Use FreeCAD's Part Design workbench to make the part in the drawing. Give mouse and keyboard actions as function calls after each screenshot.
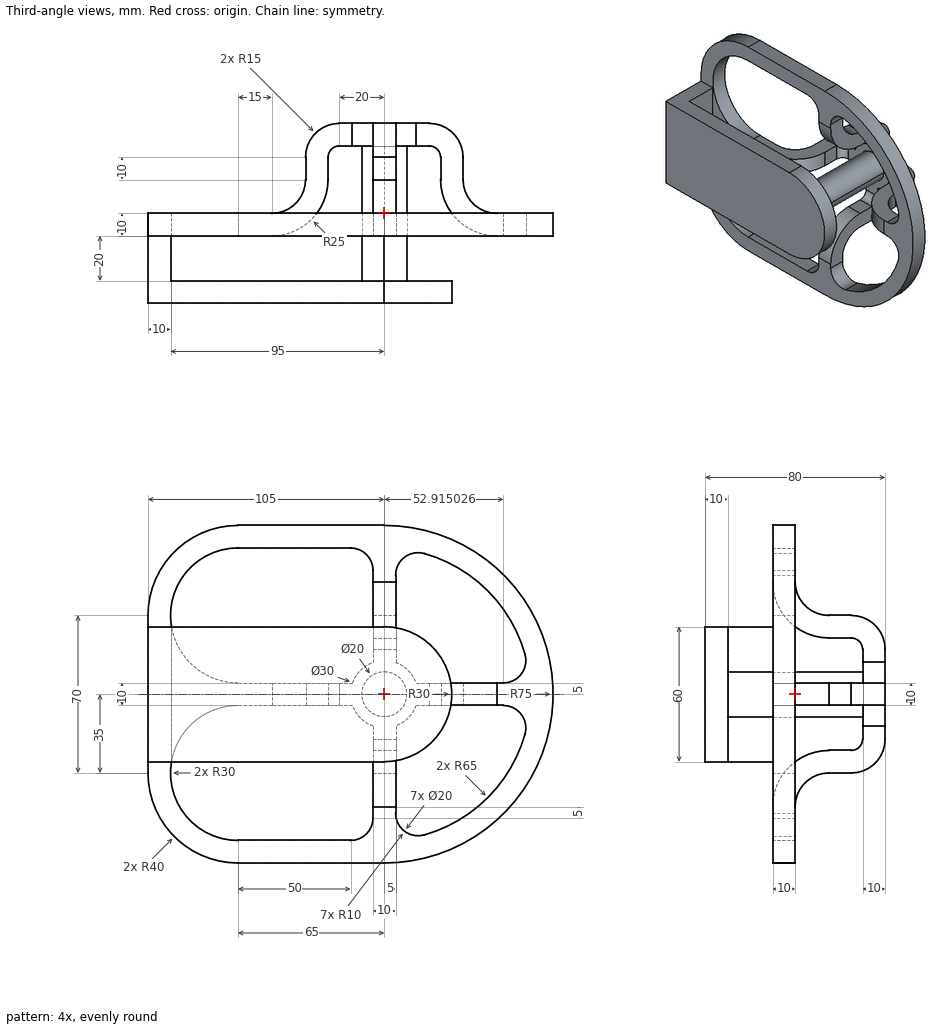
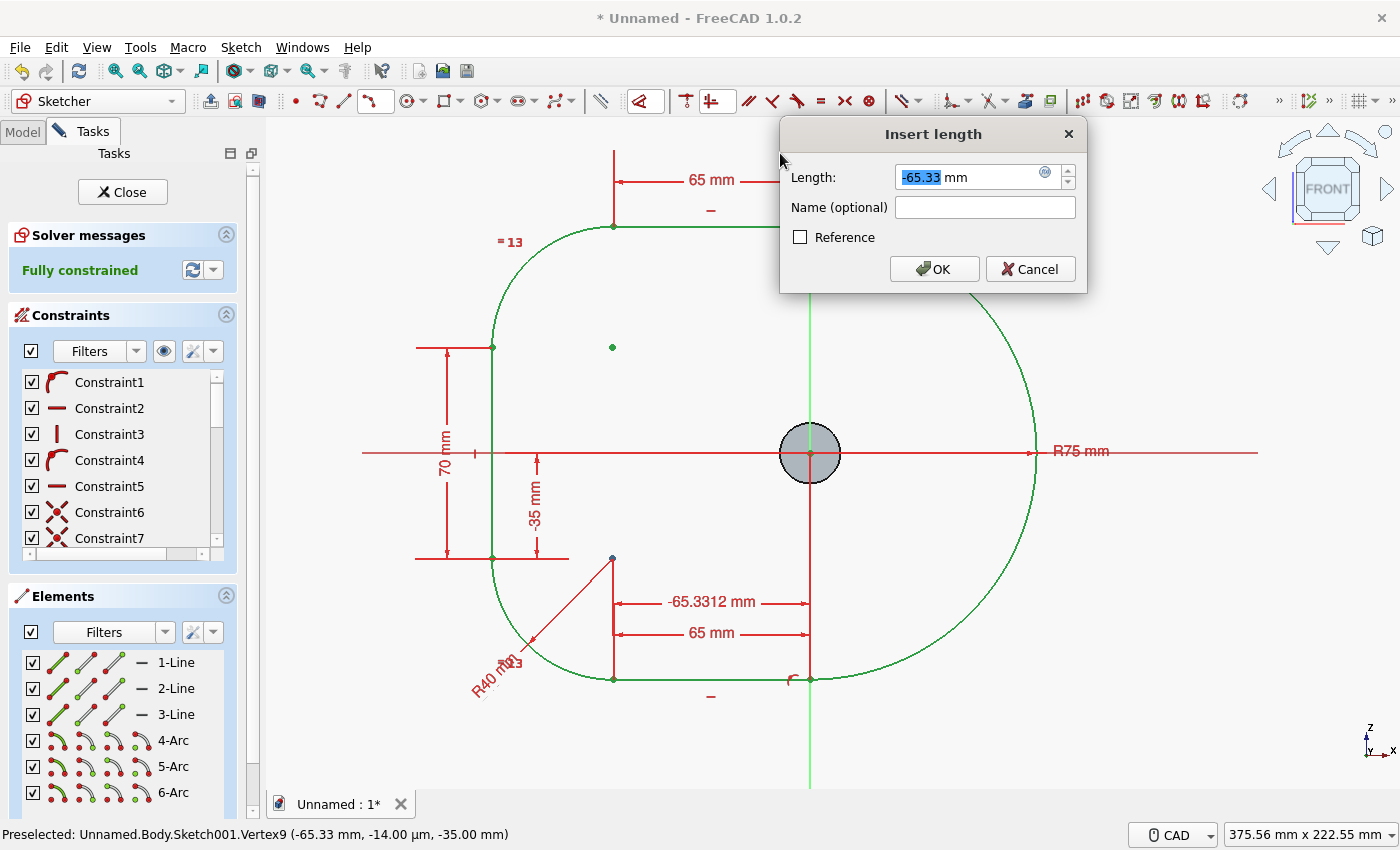
text(-65)
key(Return)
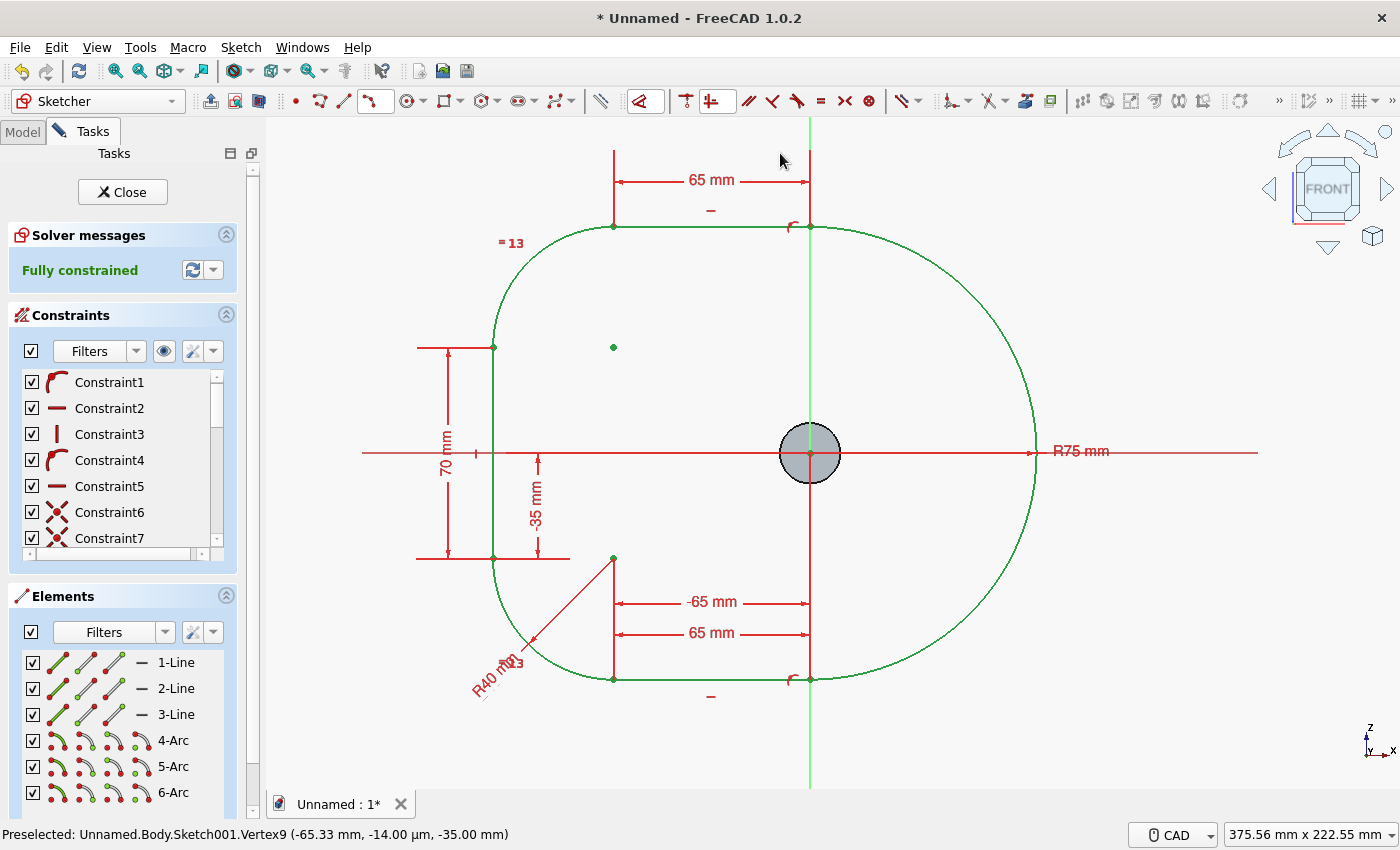
click(123, 192)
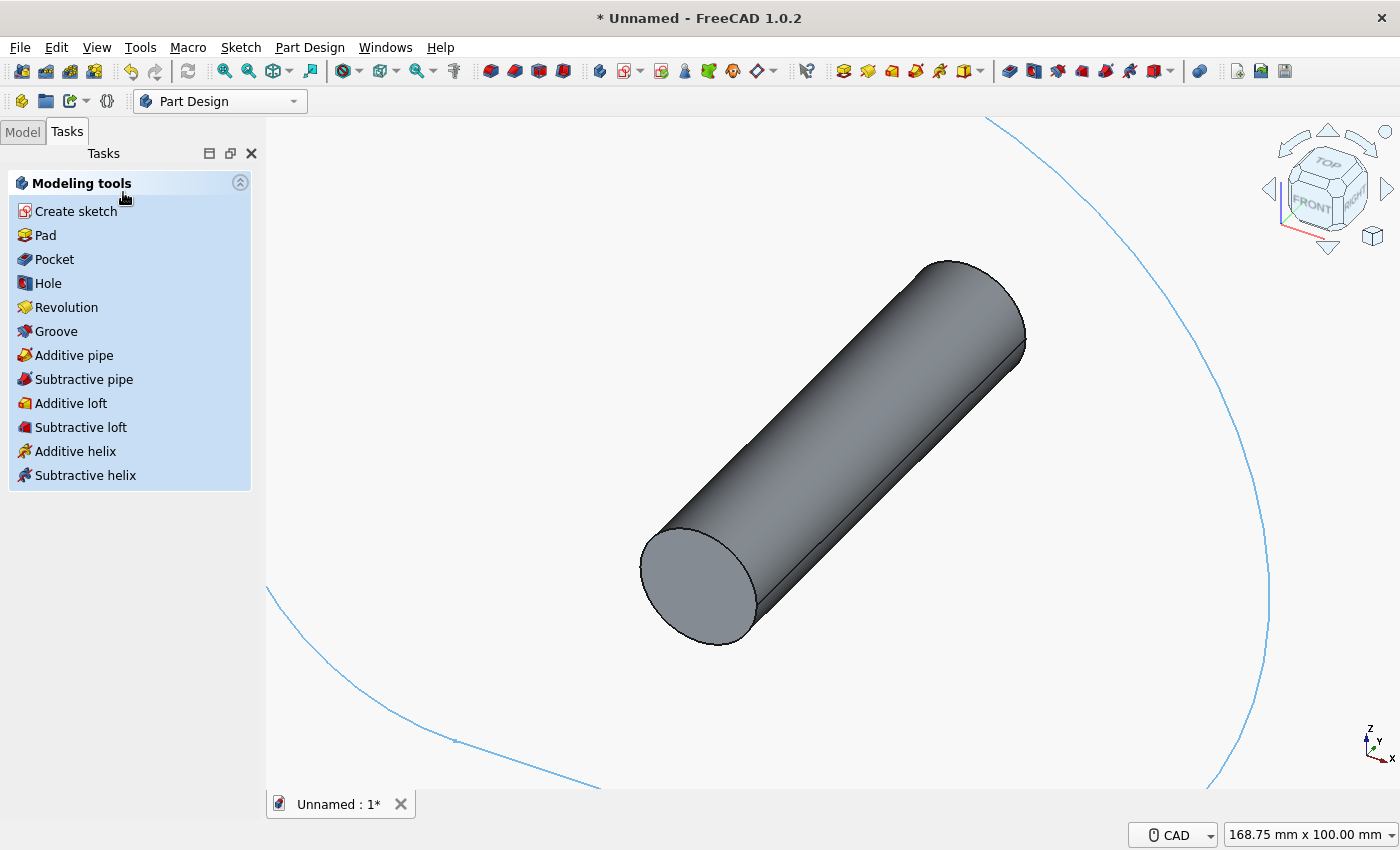
click(844, 72)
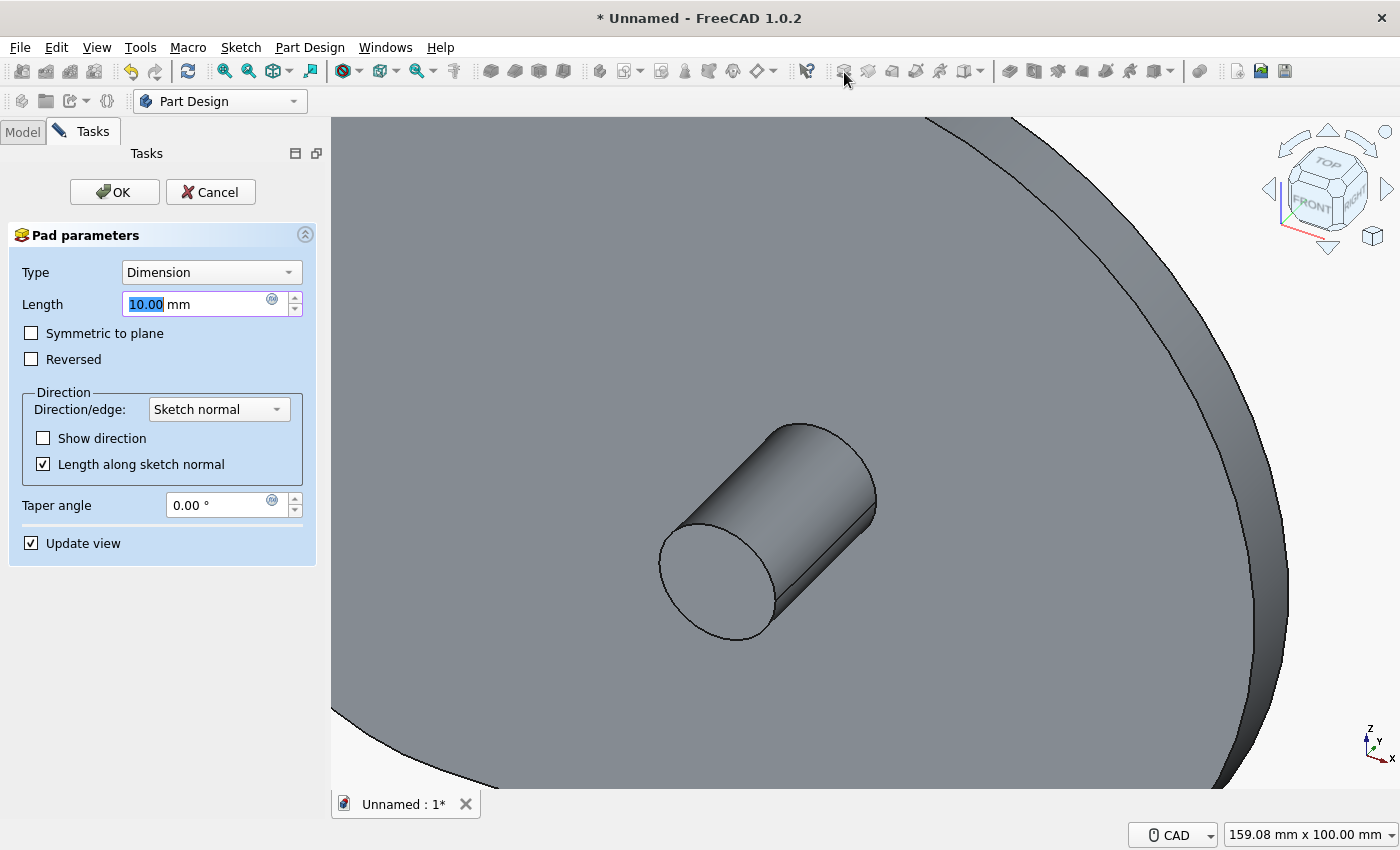
text(10)
key(Tab)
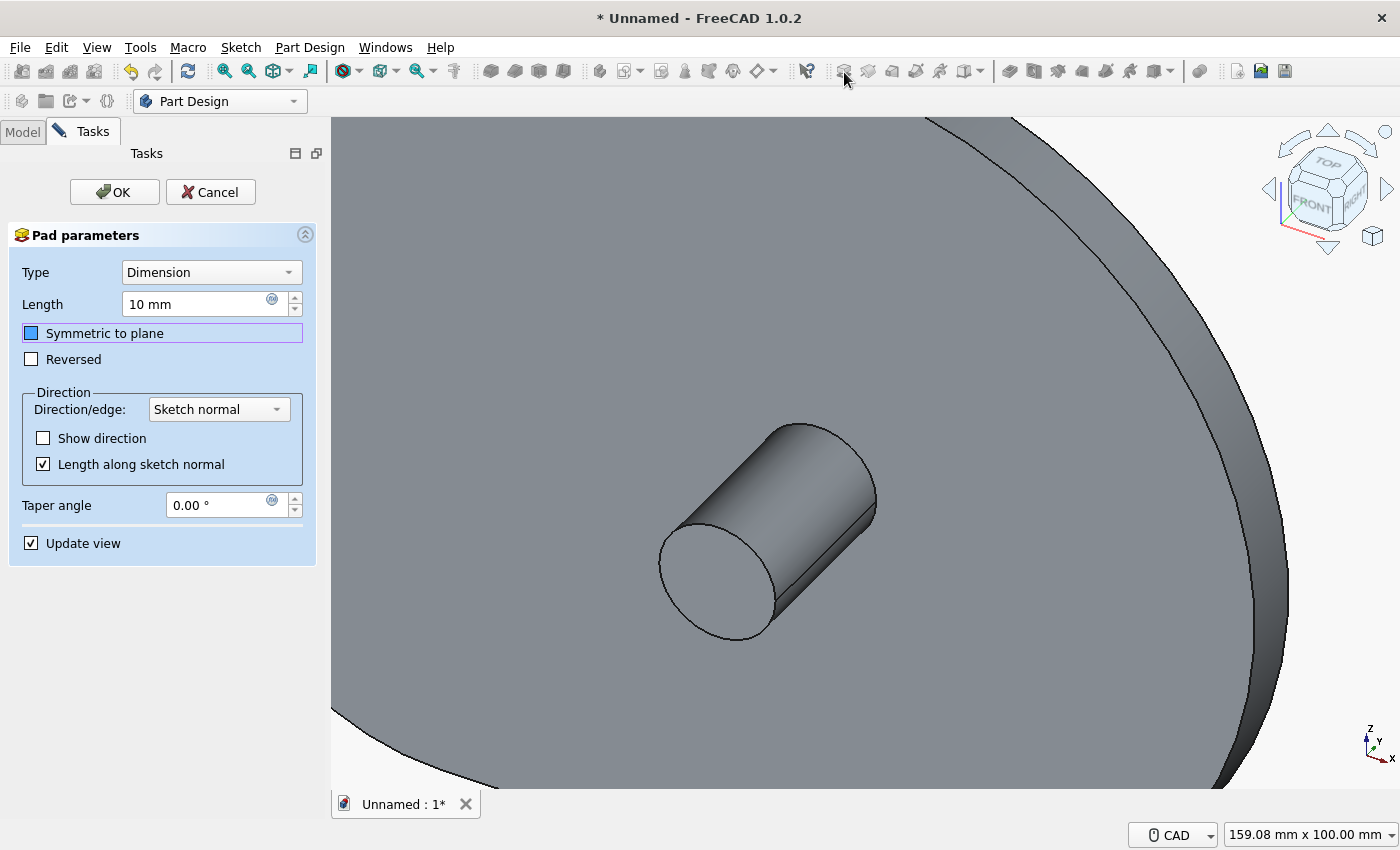
click(115, 192)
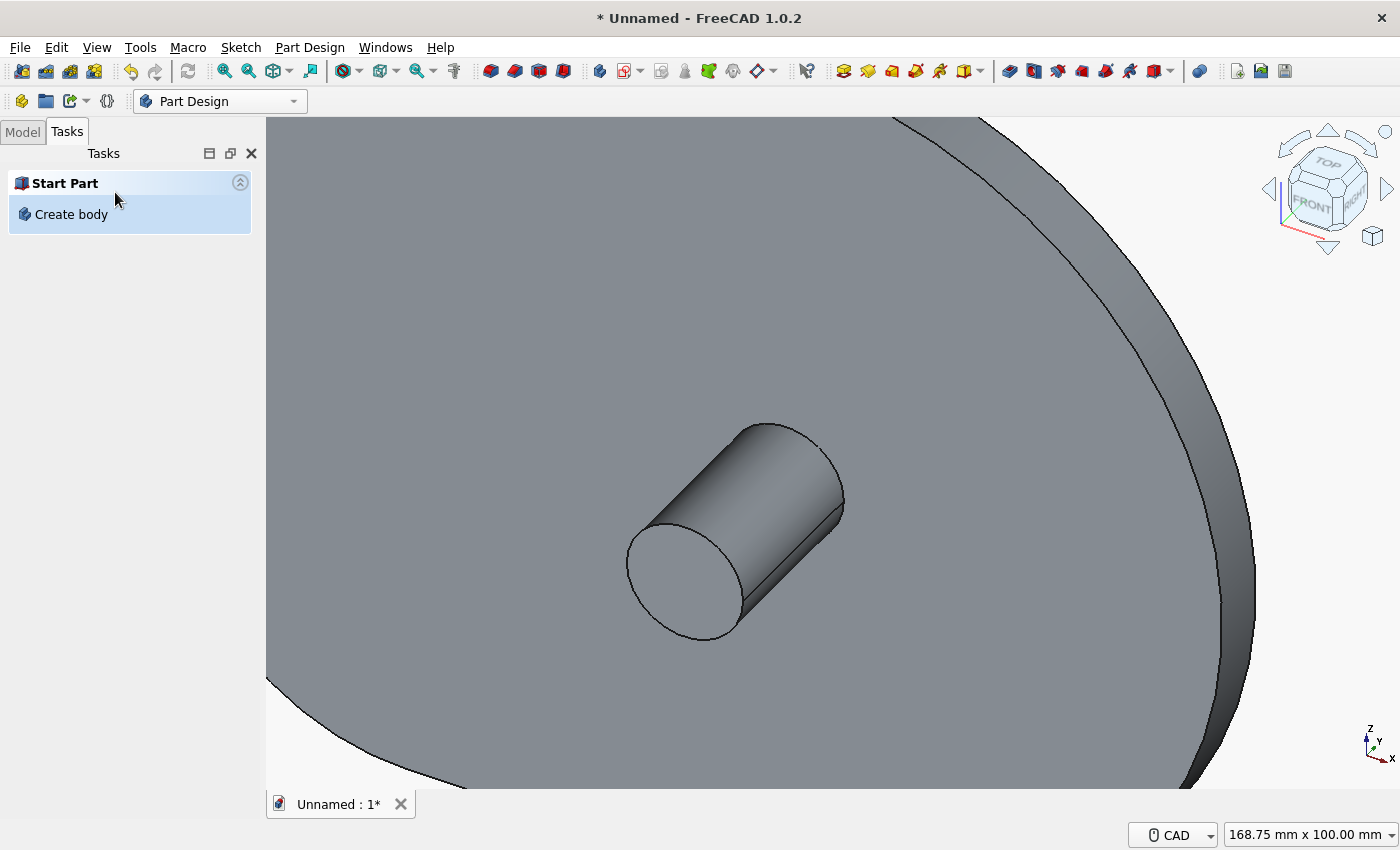
click(226, 72)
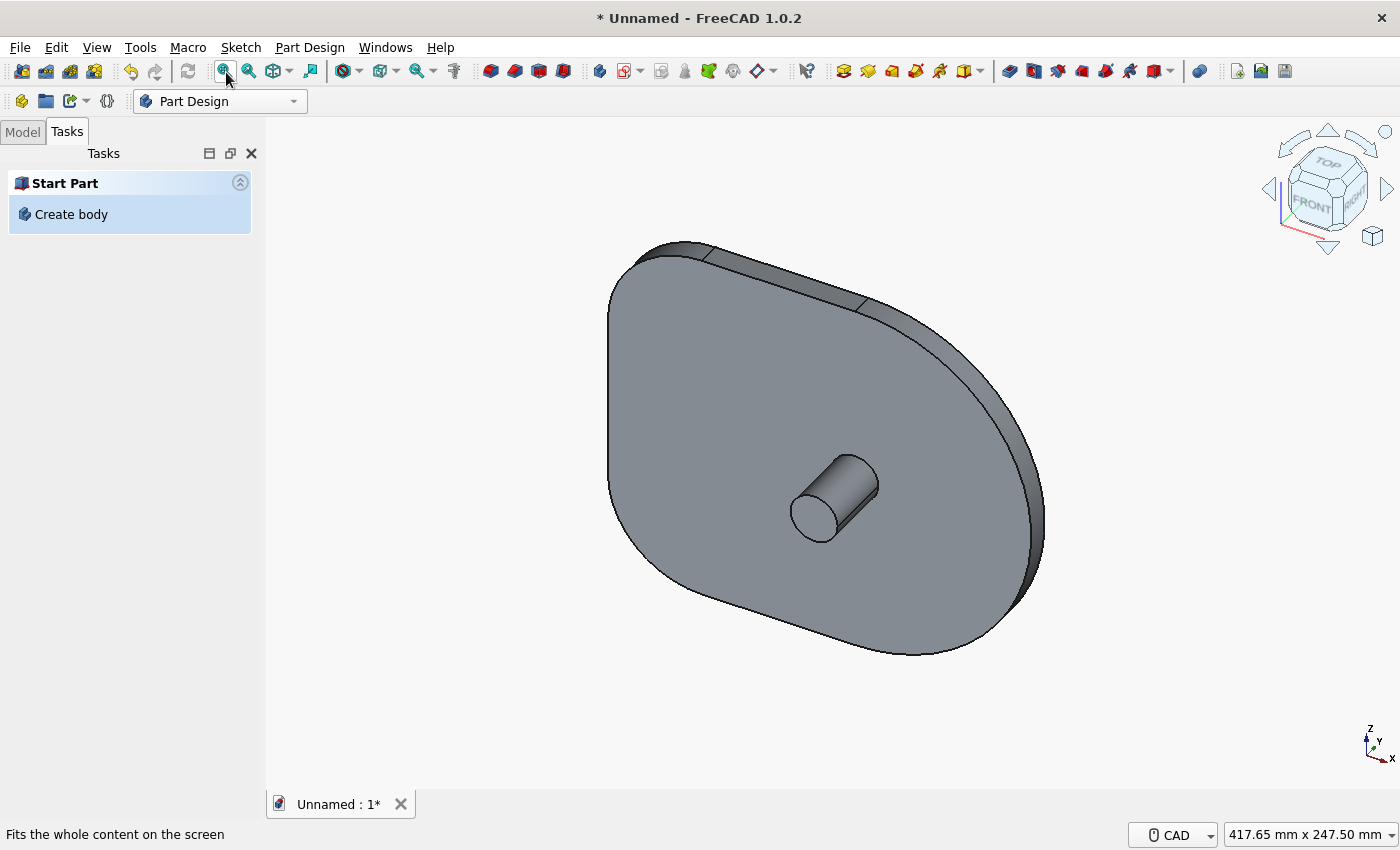
click(814, 518)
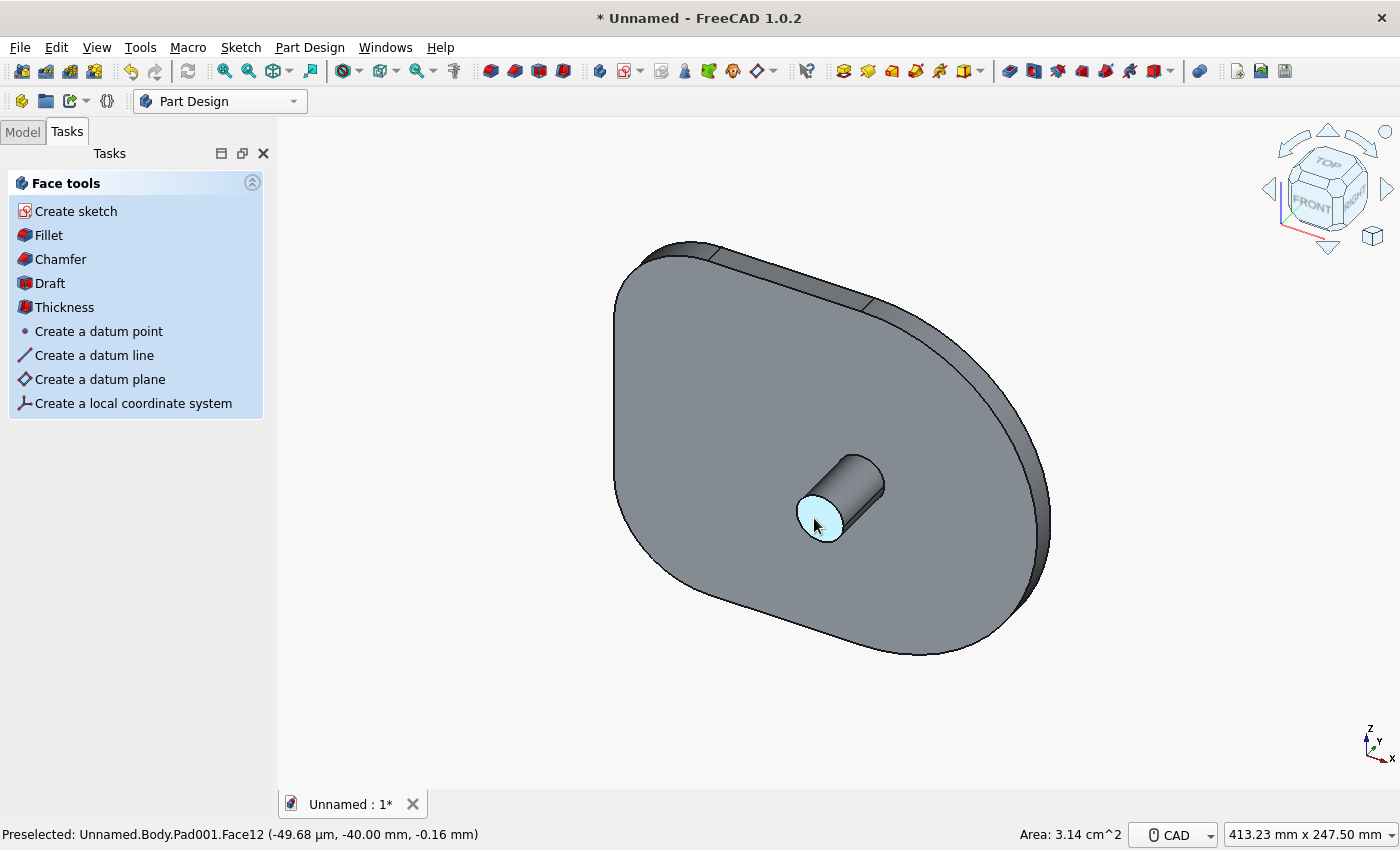
click(624, 72)